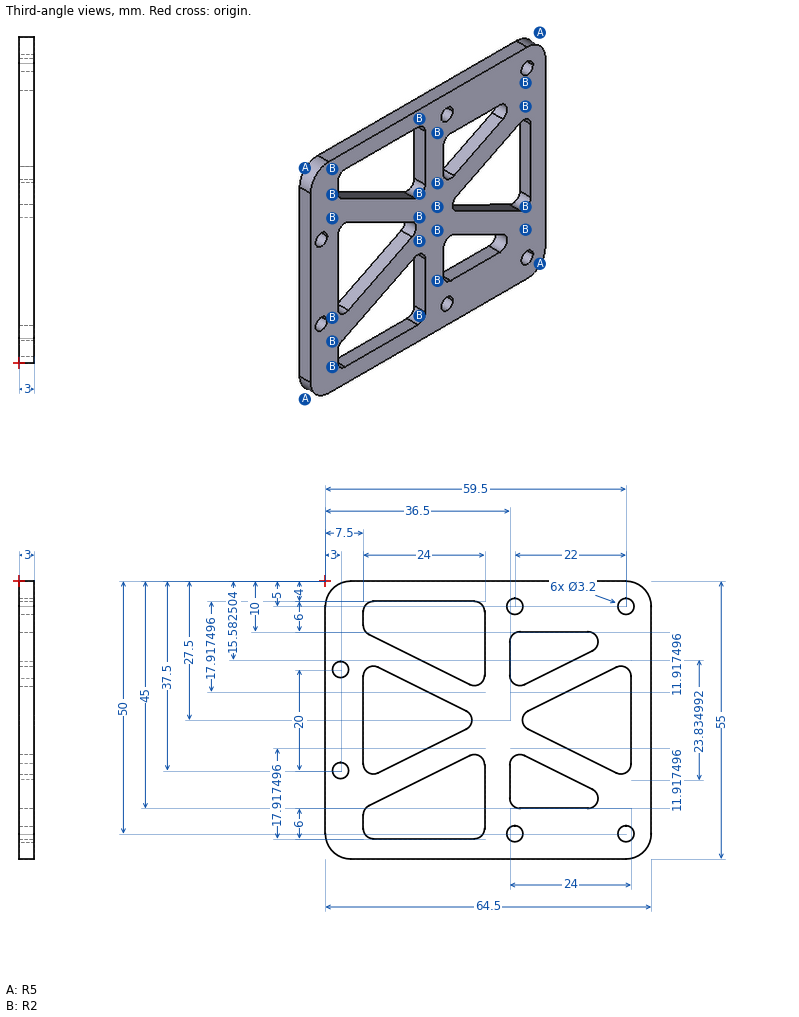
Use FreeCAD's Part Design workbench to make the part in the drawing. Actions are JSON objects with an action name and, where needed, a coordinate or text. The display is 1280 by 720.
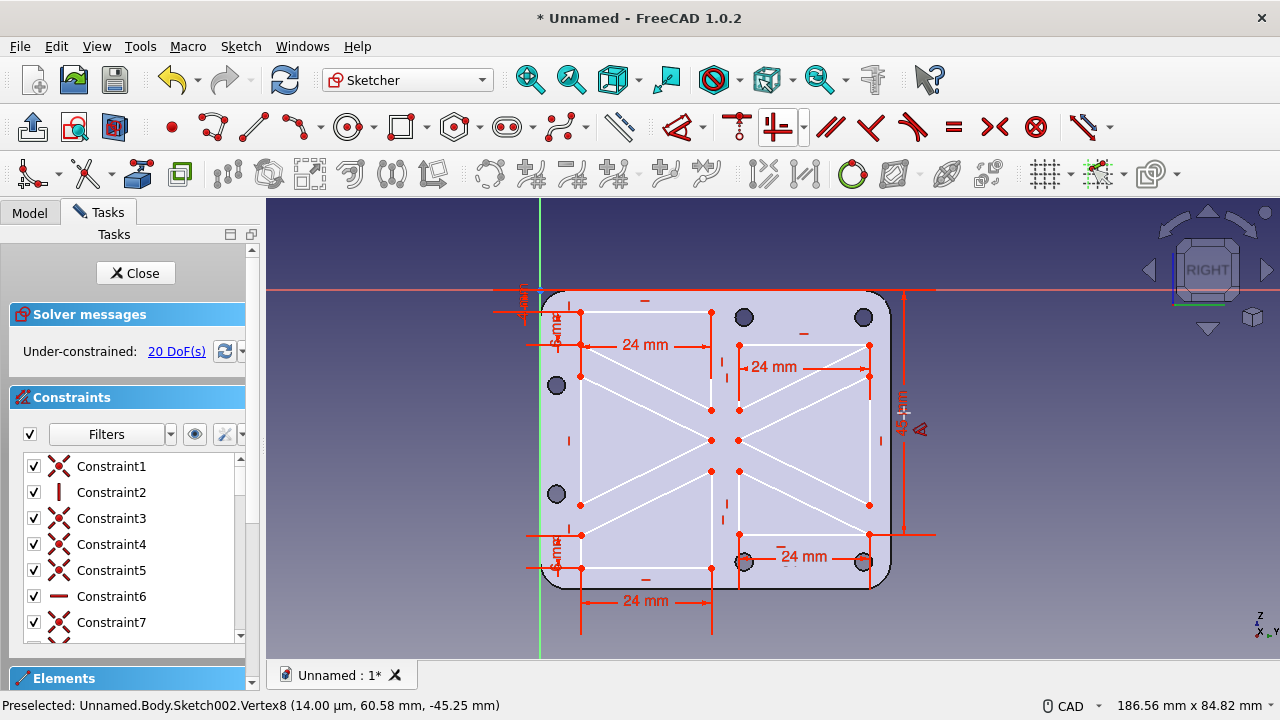
{"action": "left_click", "coordinate": [739, 345]}
{"action": "left_click", "coordinate": [773, 318]}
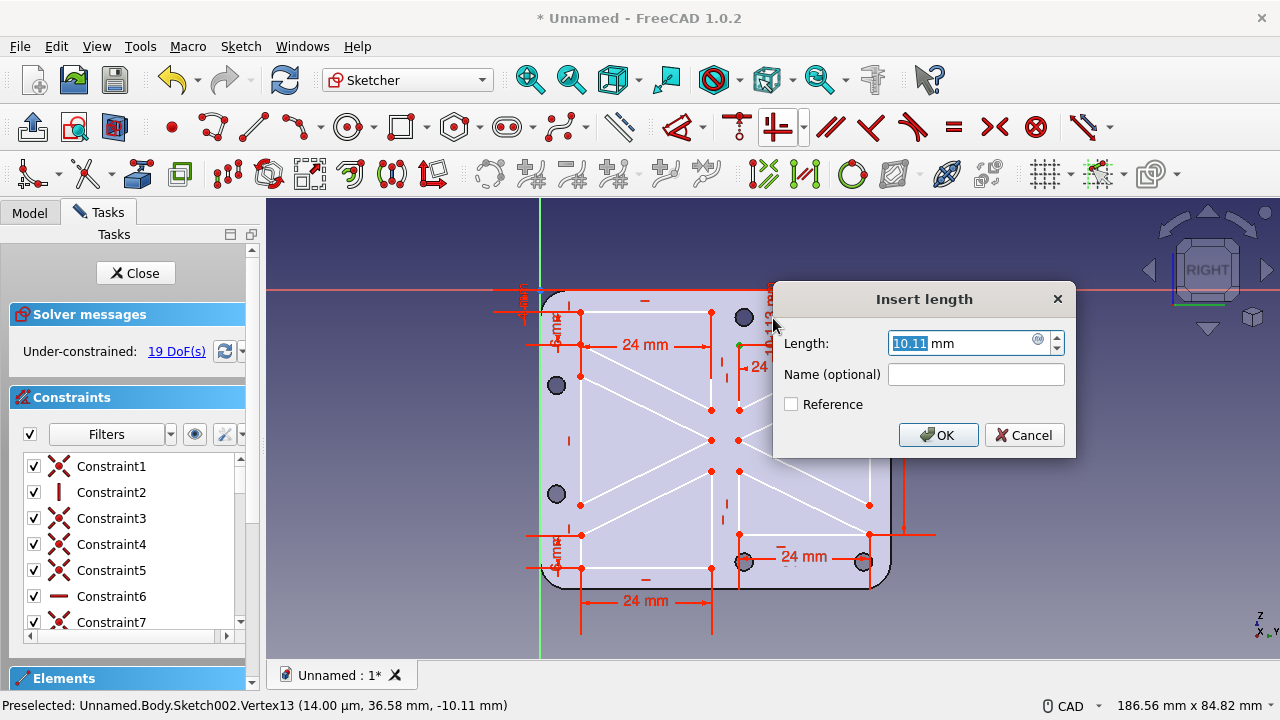
{"action": "type", "text": "10"}
{"action": "key", "text": "Return"}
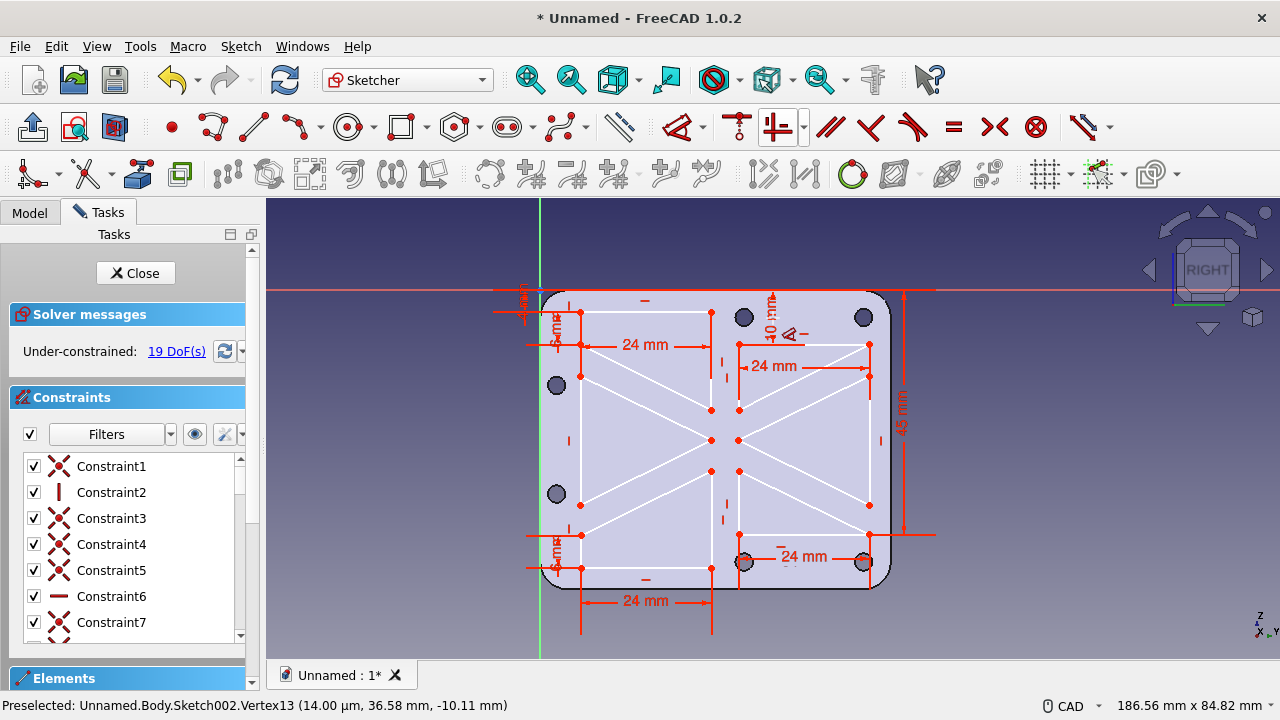
{"action": "left_click", "coordinate": [581, 536]}
{"action": "left_click", "coordinate": [506, 413]}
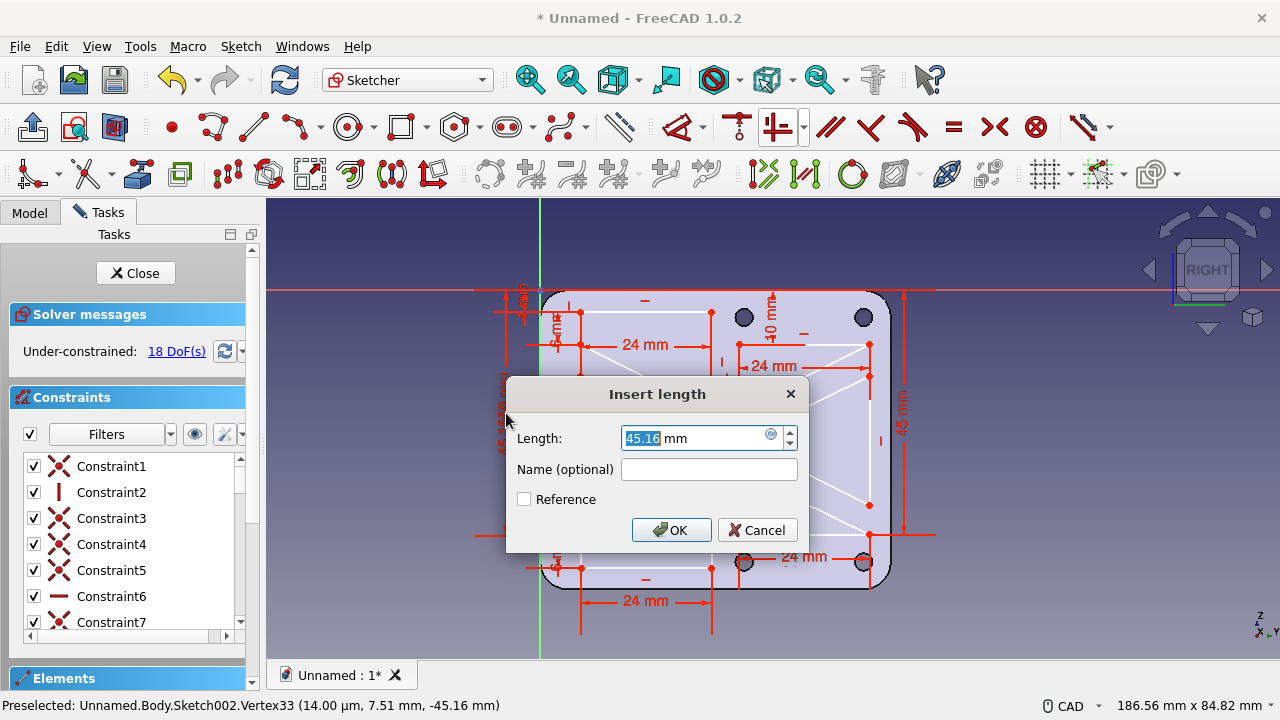
{"action": "type", "text": "45"}
{"action": "key", "text": "Return"}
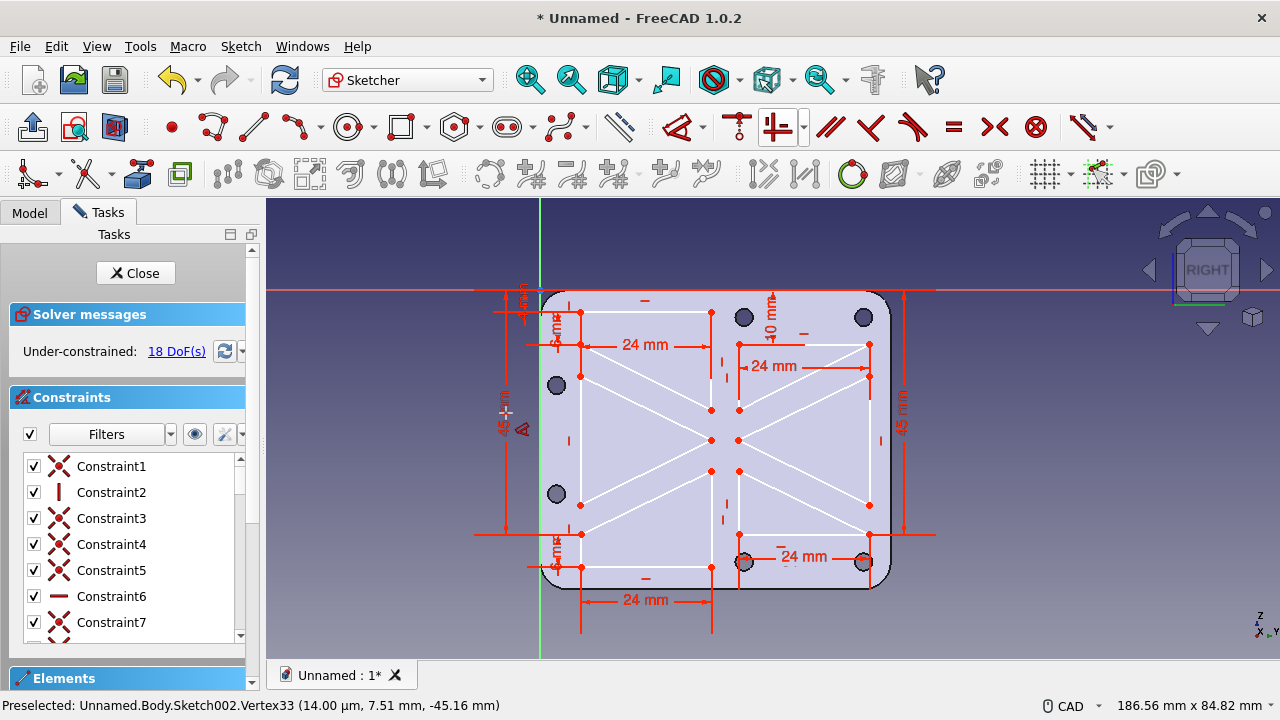
{"action": "left_click", "coordinate": [778, 421]}
{"action": "left_click", "coordinate": [850, 474]}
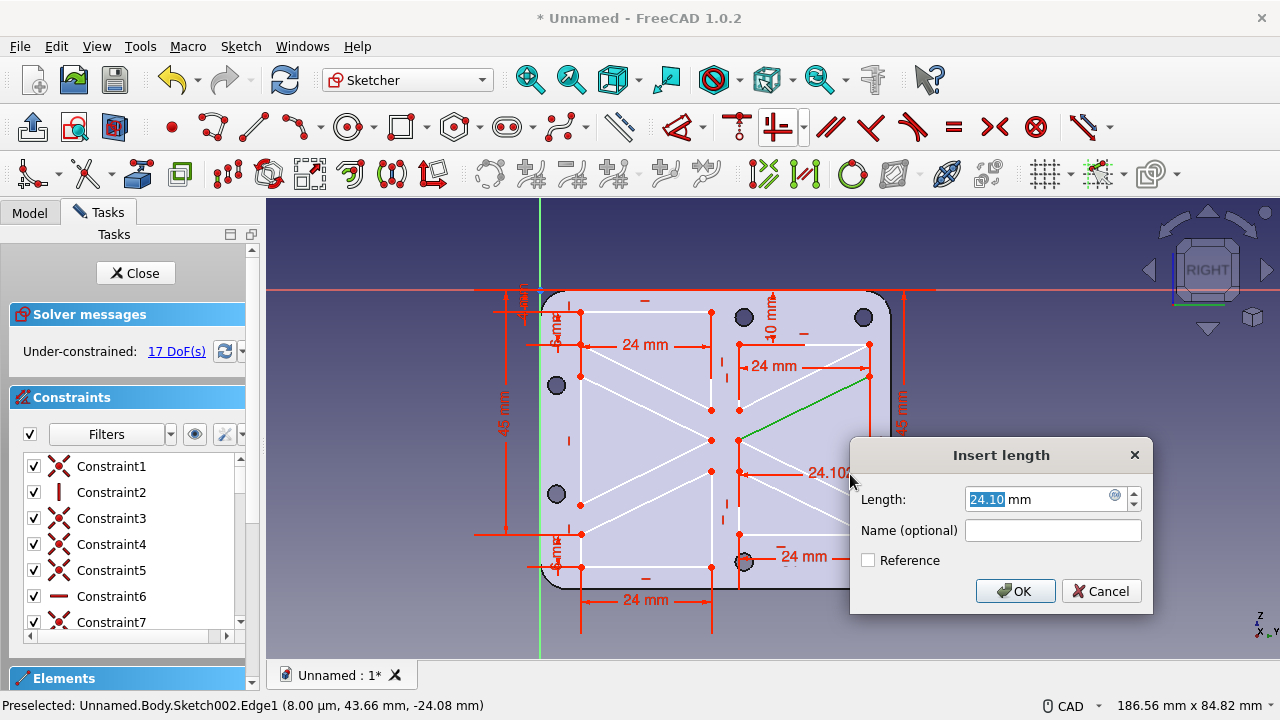
{"action": "type", "text": "24"}
{"action": "key", "text": "Return"}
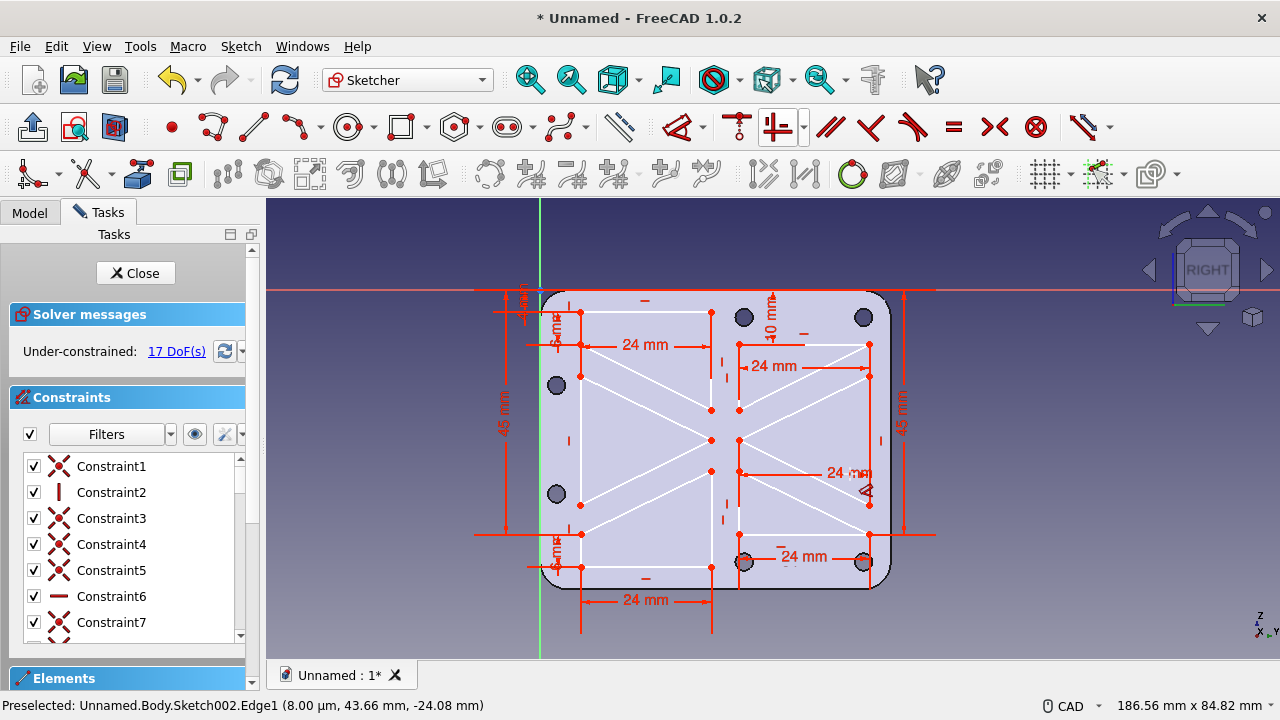
{"action": "left_click", "coordinate": [620, 395]}
{"action": "left_click", "coordinate": [600, 474]}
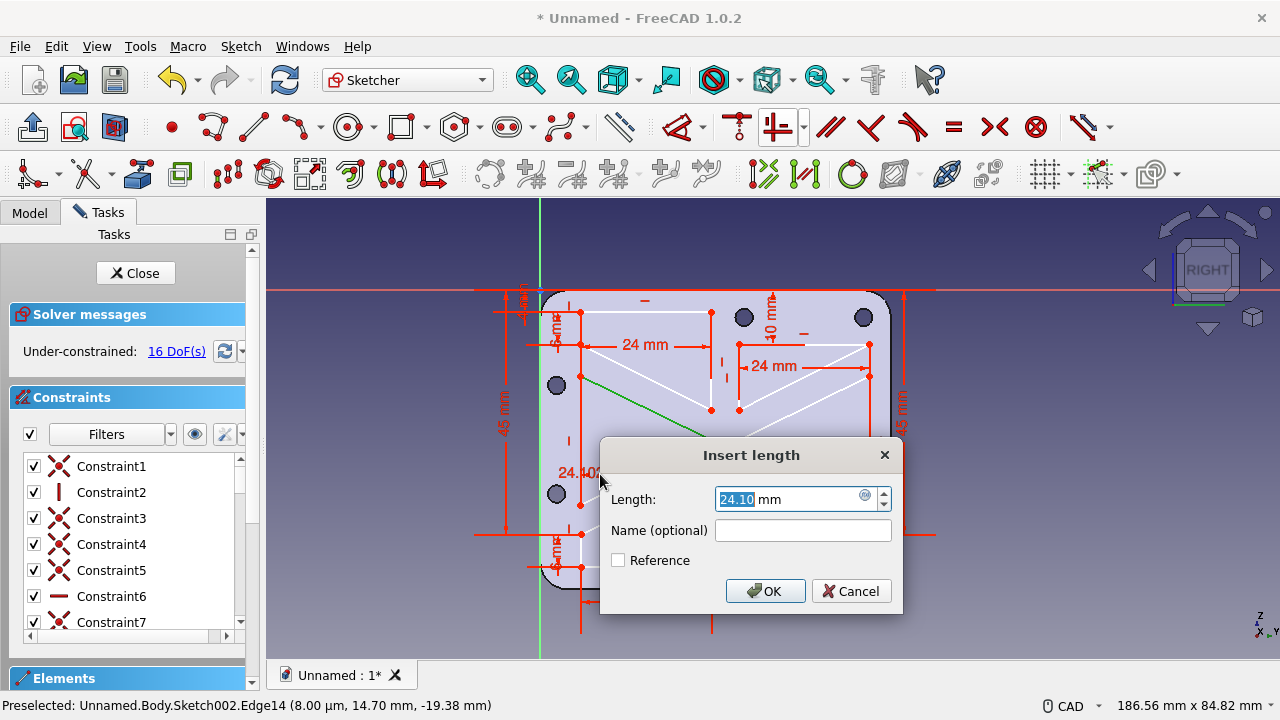
{"action": "type", "text": "24"}
{"action": "key", "text": "Return"}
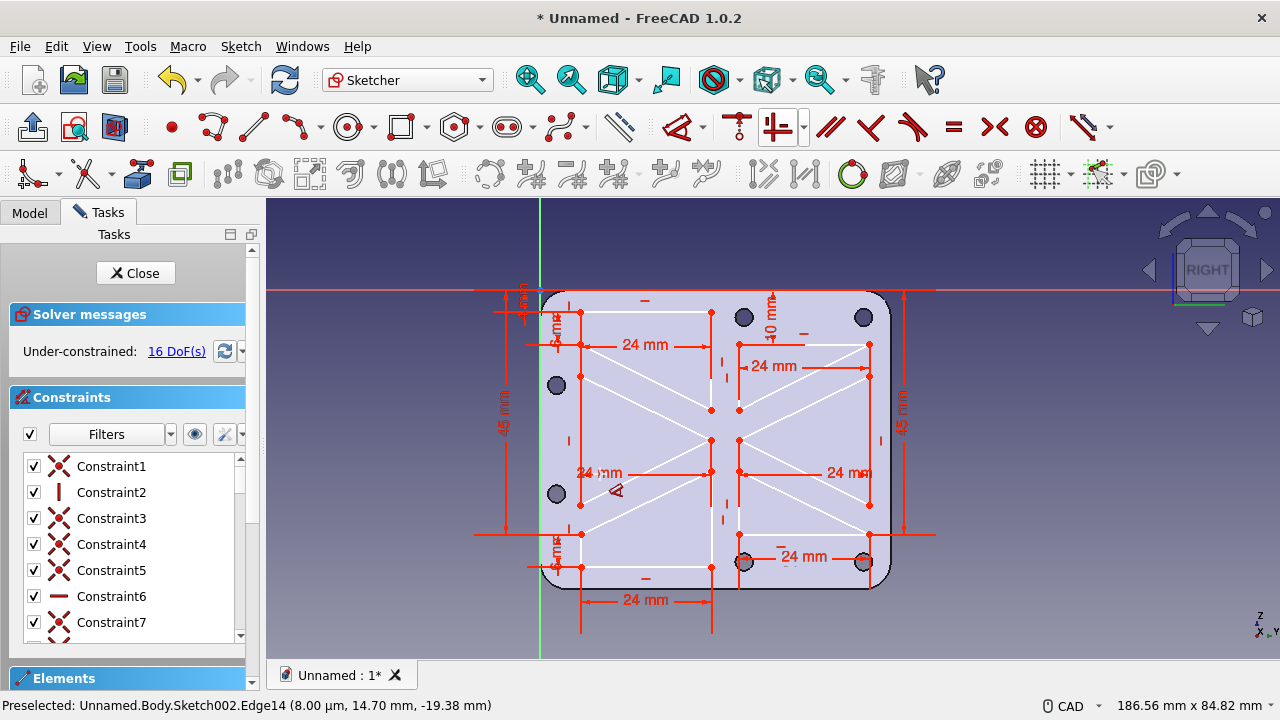
{"action": "left_click", "coordinate": [581, 312]}
{"action": "left_click", "coordinate": [560, 256]}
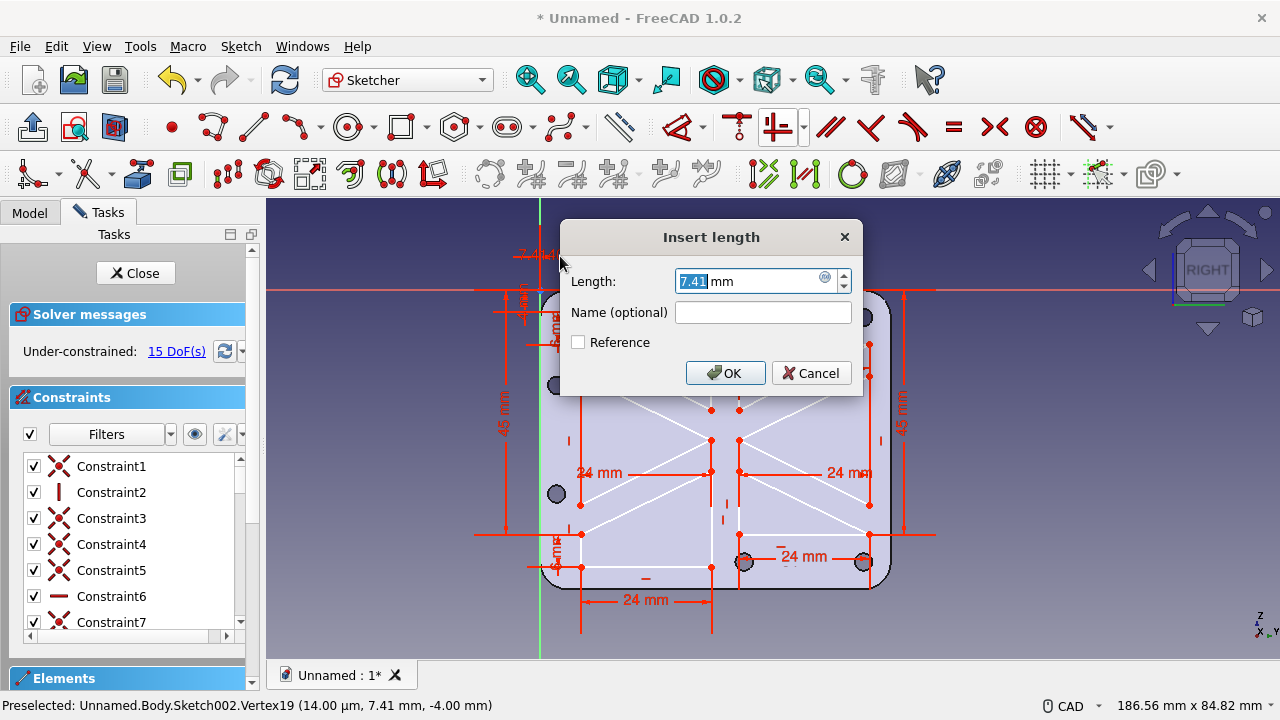
{"action": "type", "text": "7.5"}
{"action": "key", "text": "Return"}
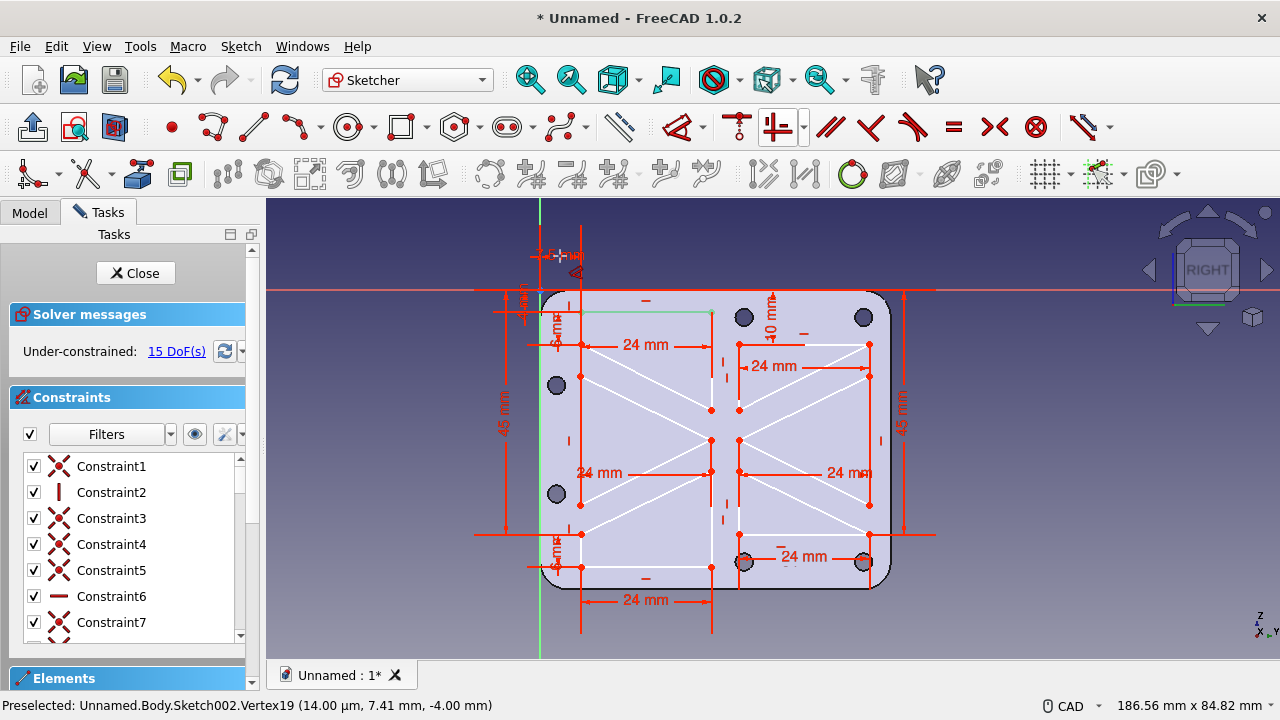
{"action": "left_click", "coordinate": [581, 376]}
{"action": "left_click", "coordinate": [560, 232]}